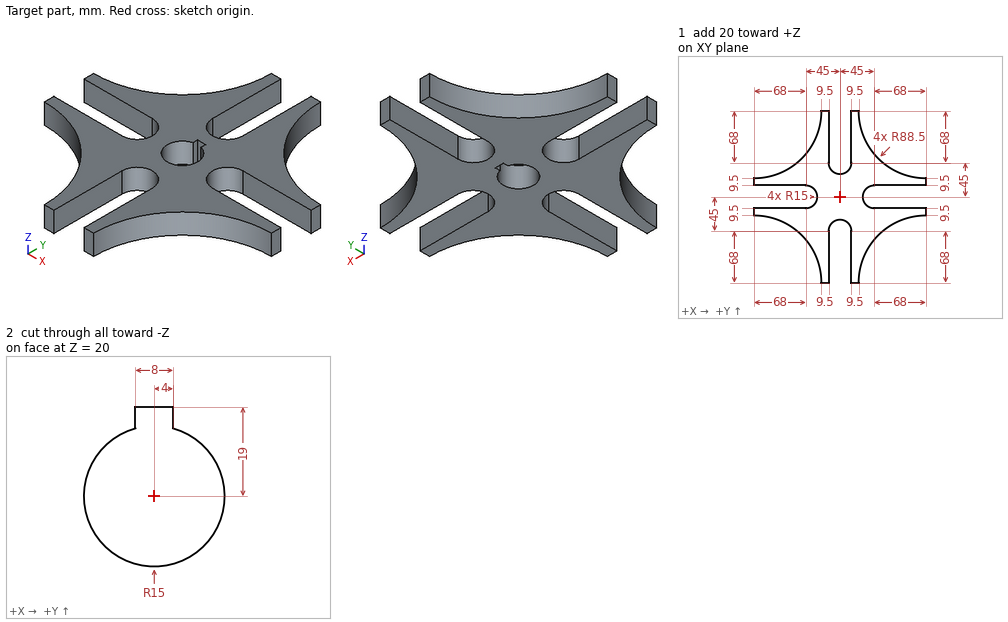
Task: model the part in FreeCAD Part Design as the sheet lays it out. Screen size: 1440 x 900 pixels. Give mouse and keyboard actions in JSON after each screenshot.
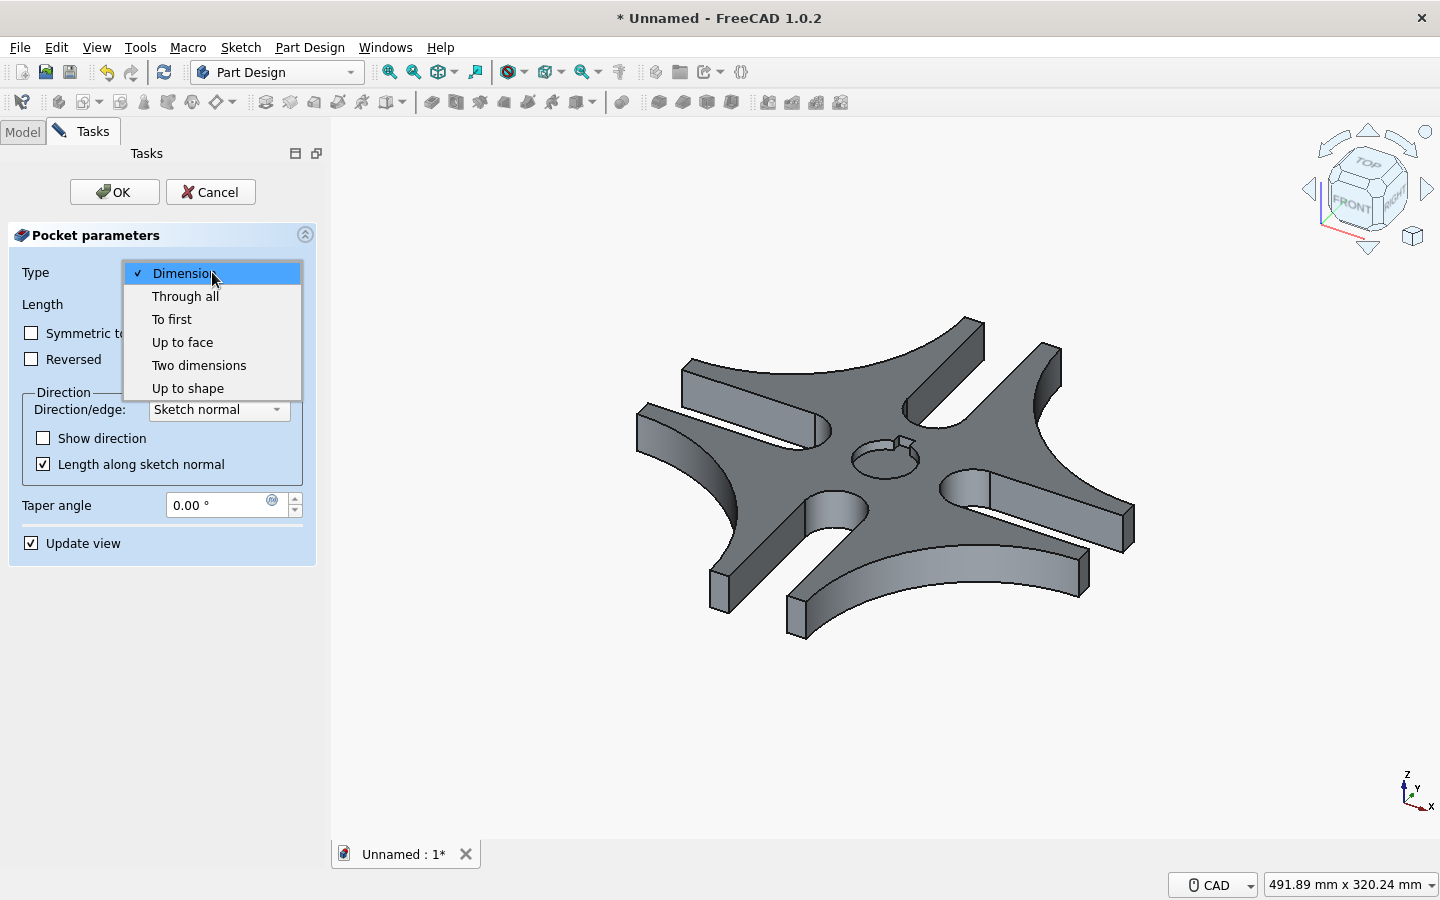
{"action": "left_click", "coordinate": [212, 296]}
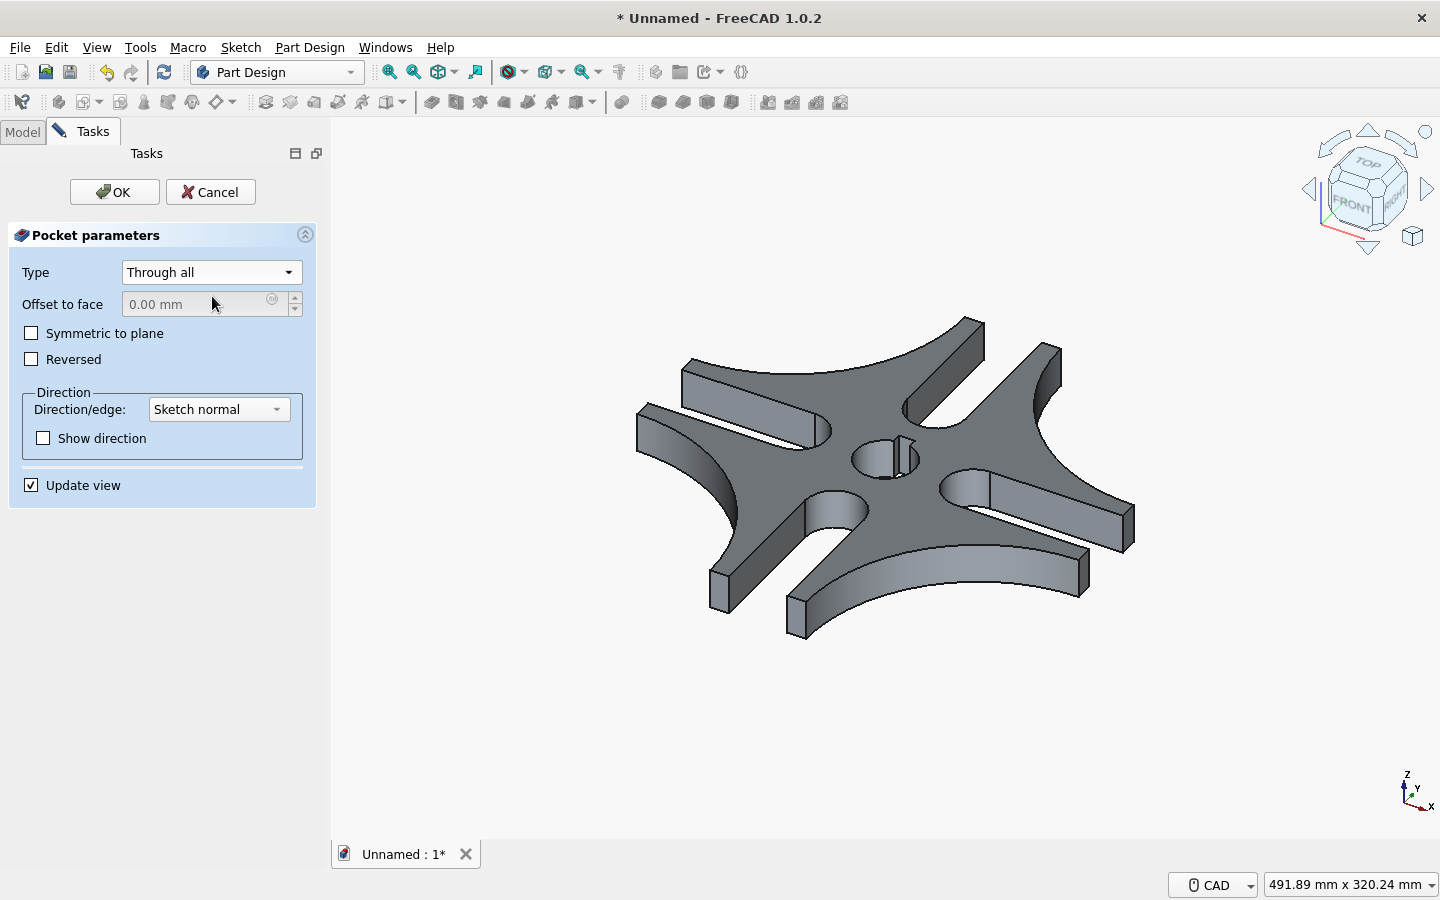
{"action": "left_click", "coordinate": [115, 192]}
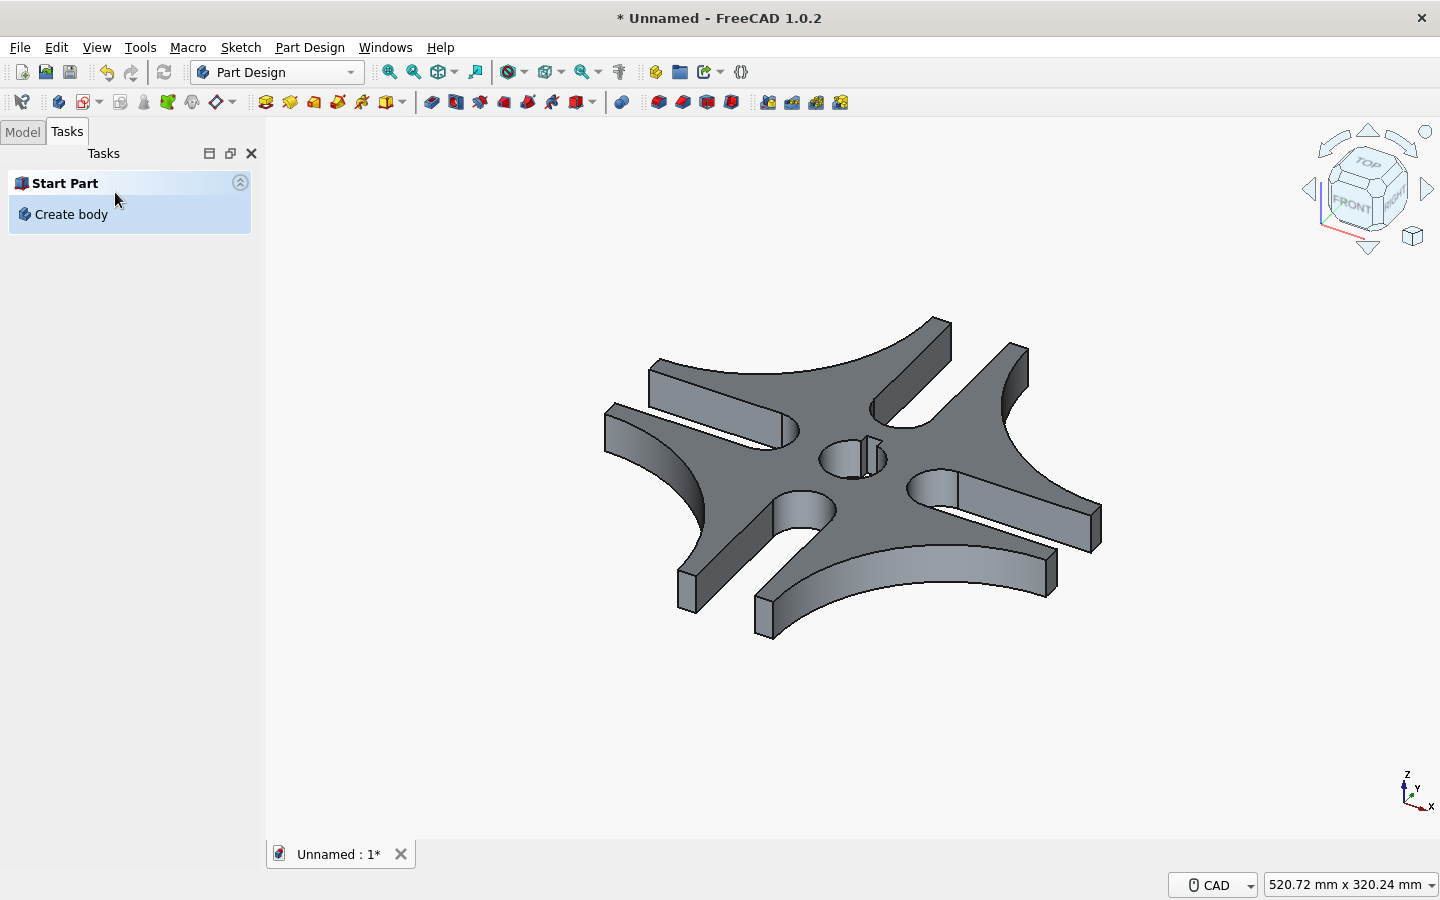
{"action": "key", "text": "0"}